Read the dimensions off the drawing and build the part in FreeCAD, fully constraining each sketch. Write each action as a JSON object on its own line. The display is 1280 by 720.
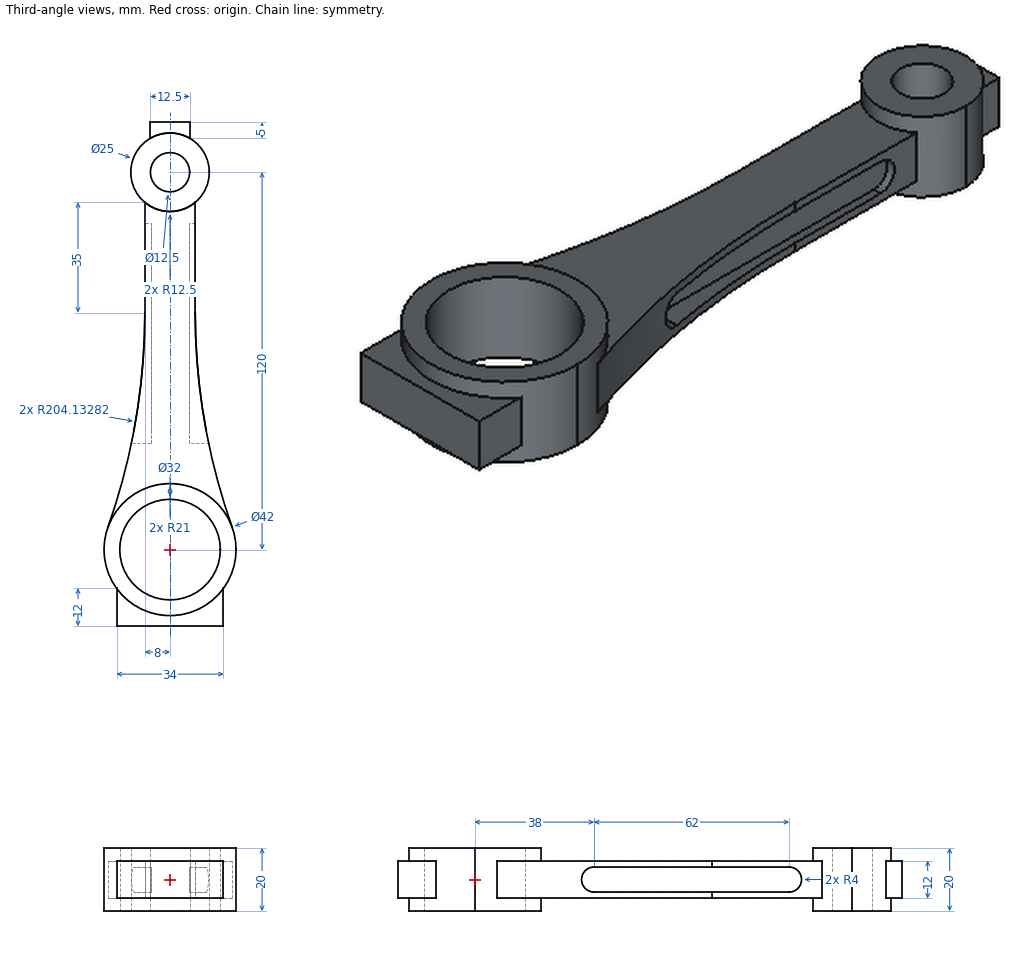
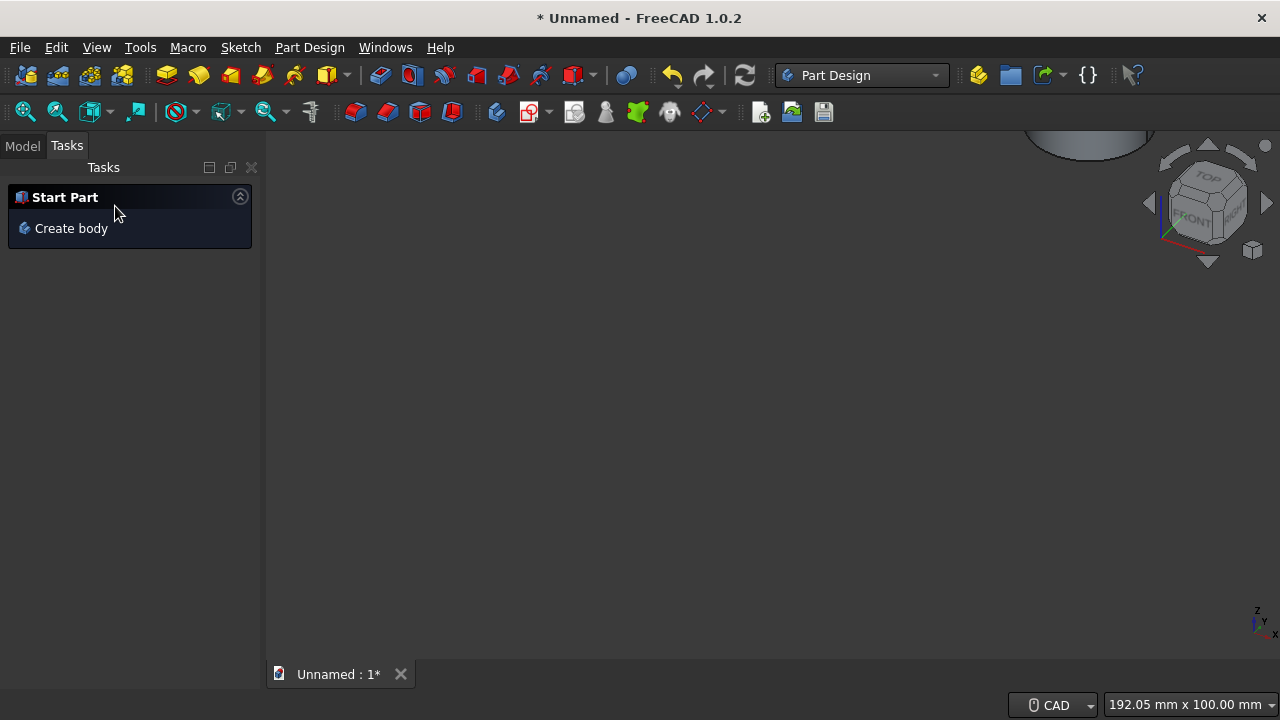
{"action": "key", "text": "v f"}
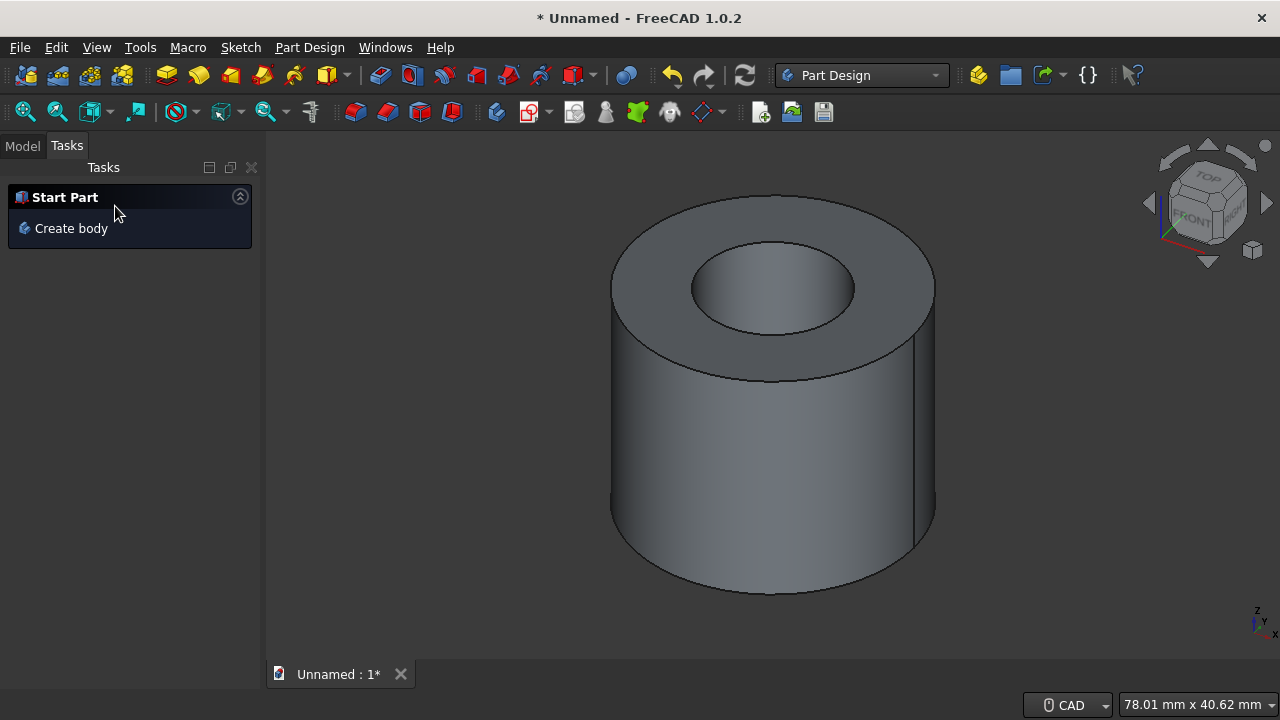
{"action": "left_click", "coordinate": [498, 112]}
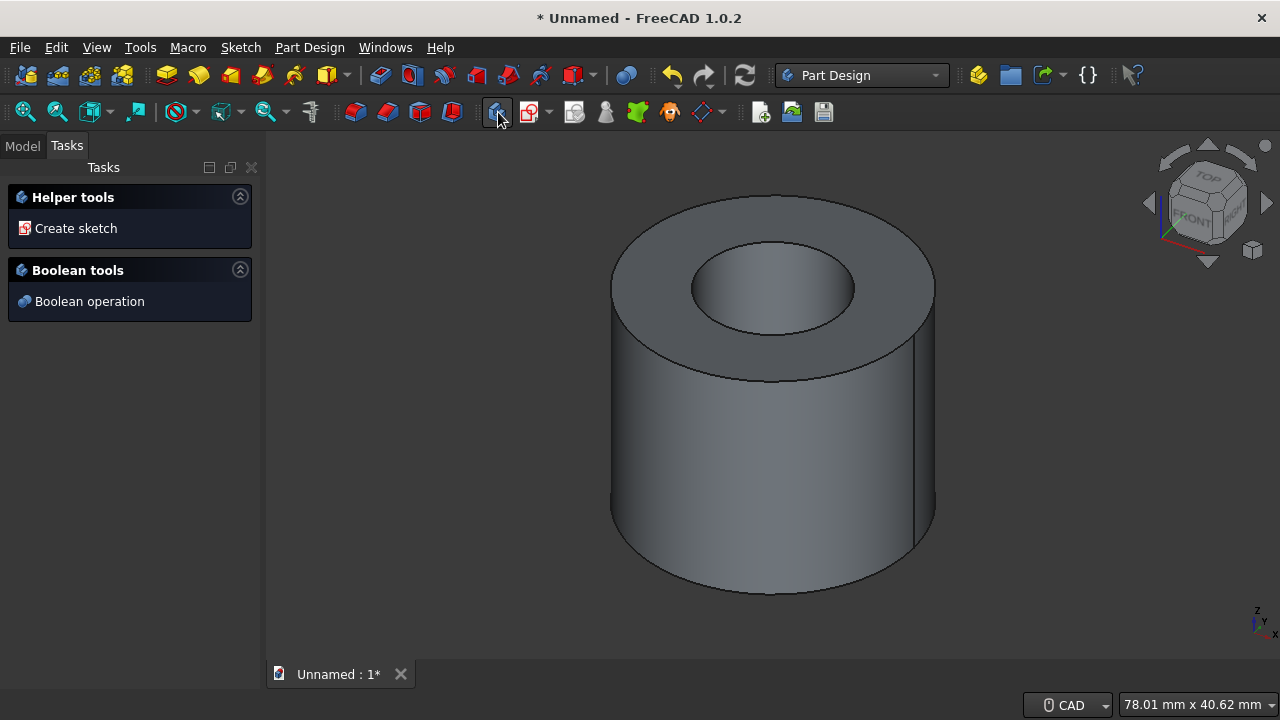
{"action": "left_click", "coordinate": [306, 619]}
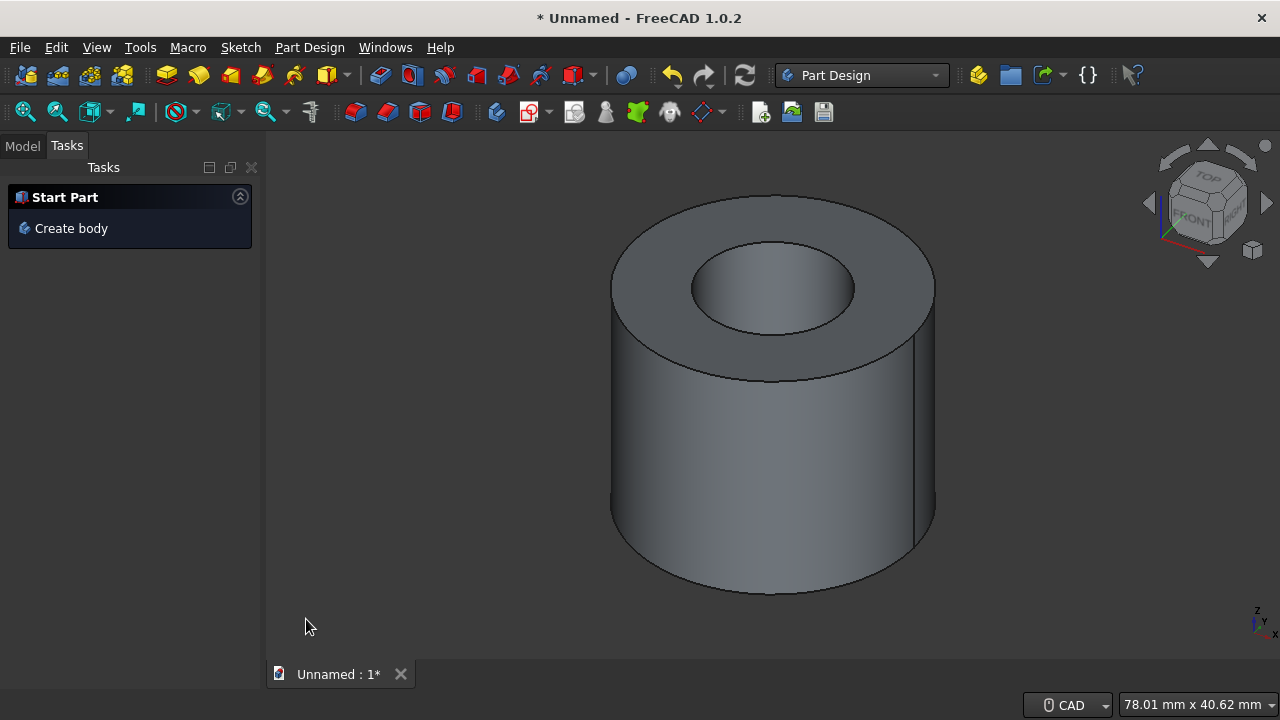
{"action": "left_click", "coordinate": [530, 112]}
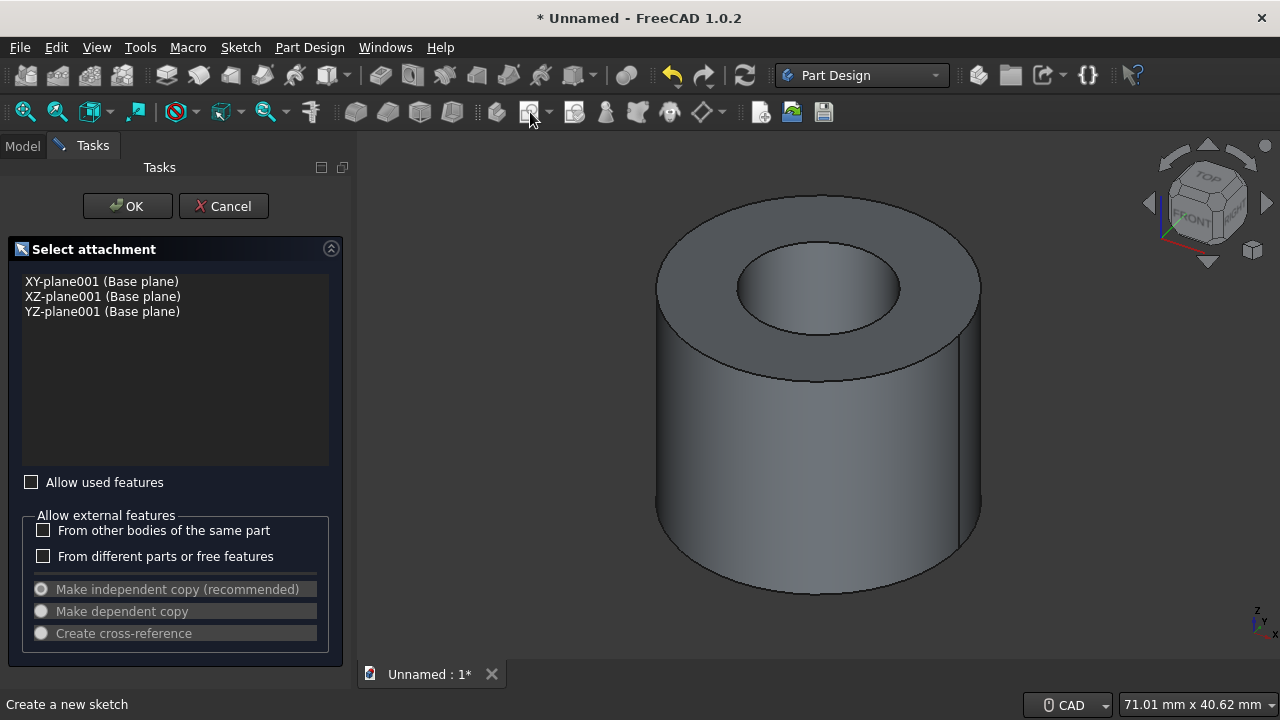
{"action": "left_click", "coordinate": [82, 282]}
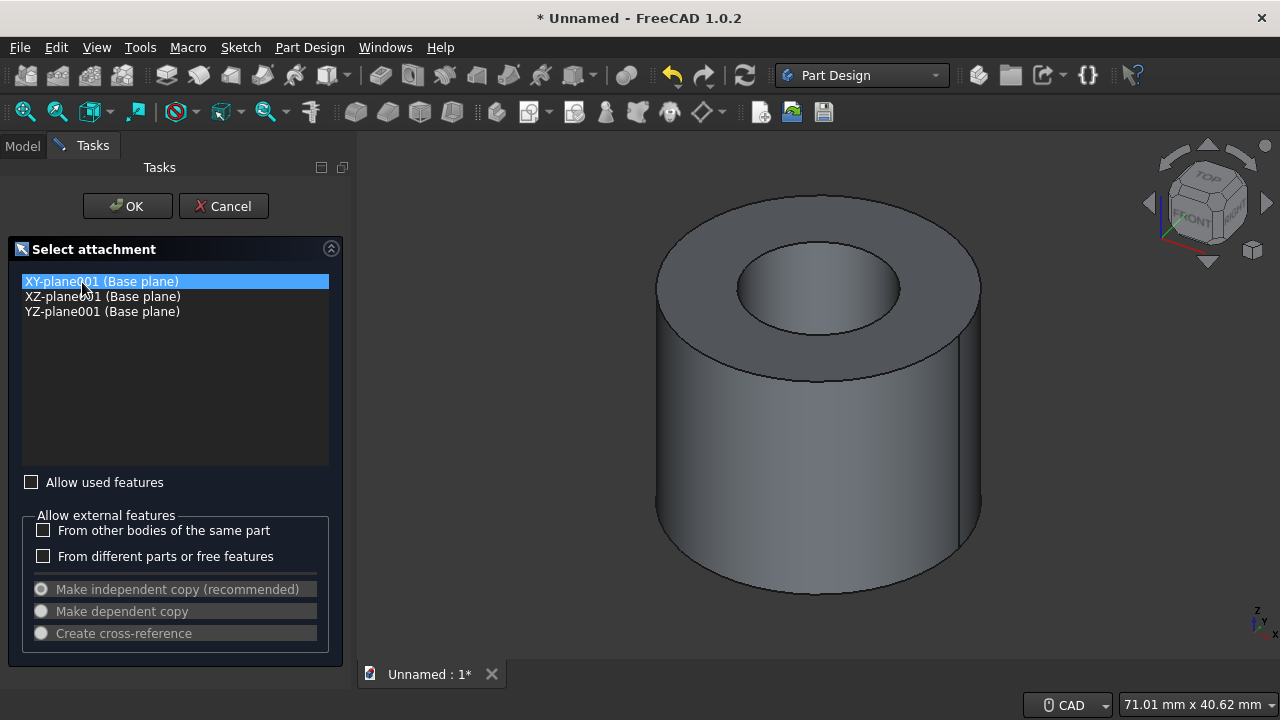
{"action": "left_click", "coordinate": [128, 206]}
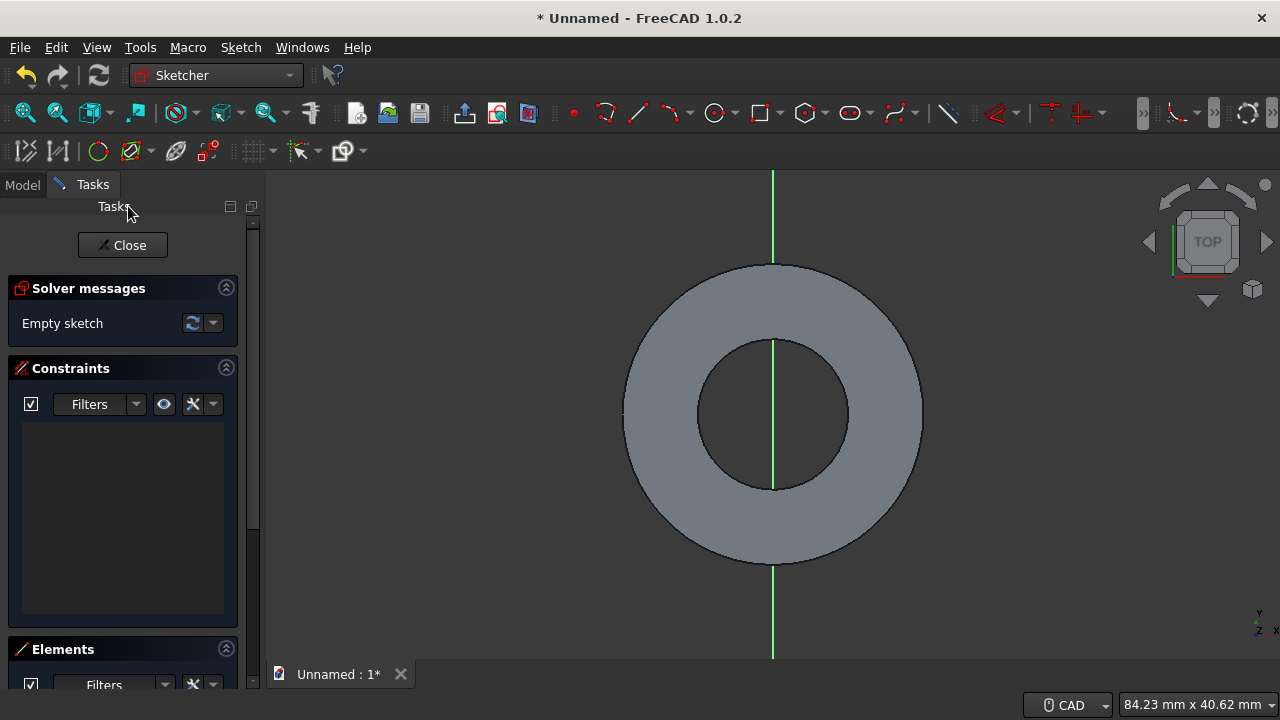
{"action": "scroll", "coordinate": [704, 414], "scroll_direction": "down", "scroll_amount": 5}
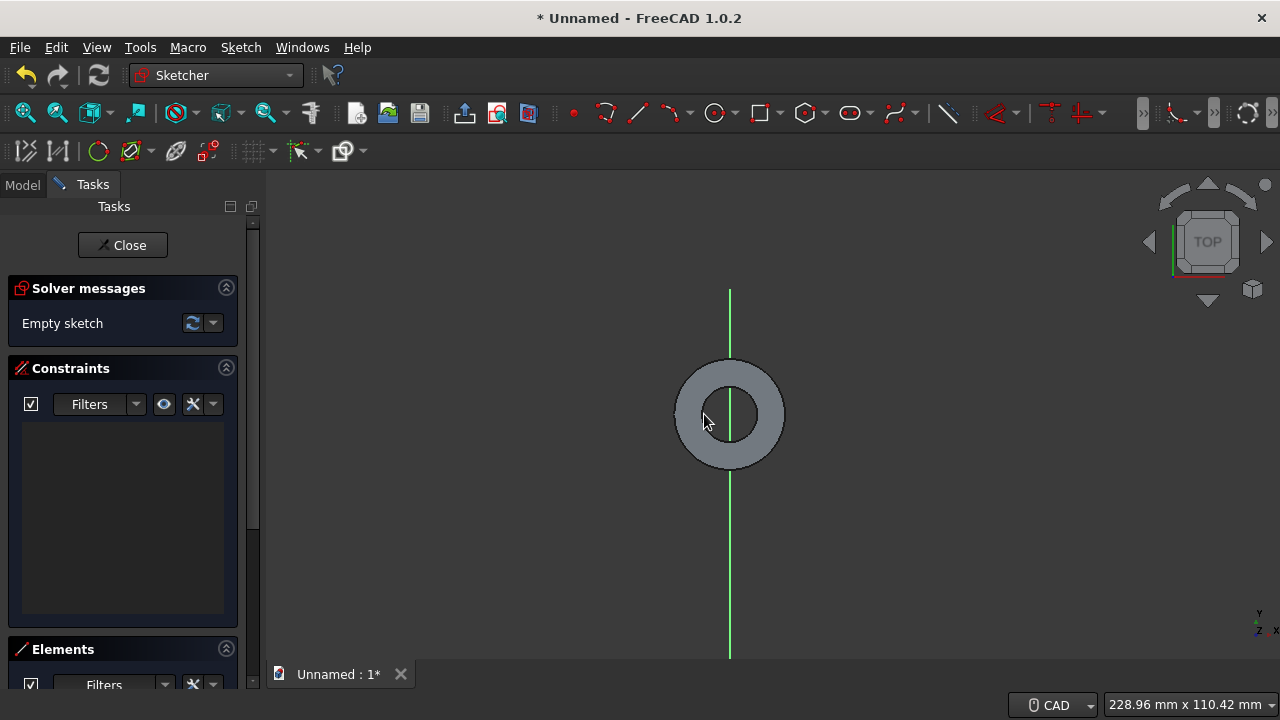
{"action": "scroll", "coordinate": [704, 414], "scroll_direction": "down", "scroll_amount": 5}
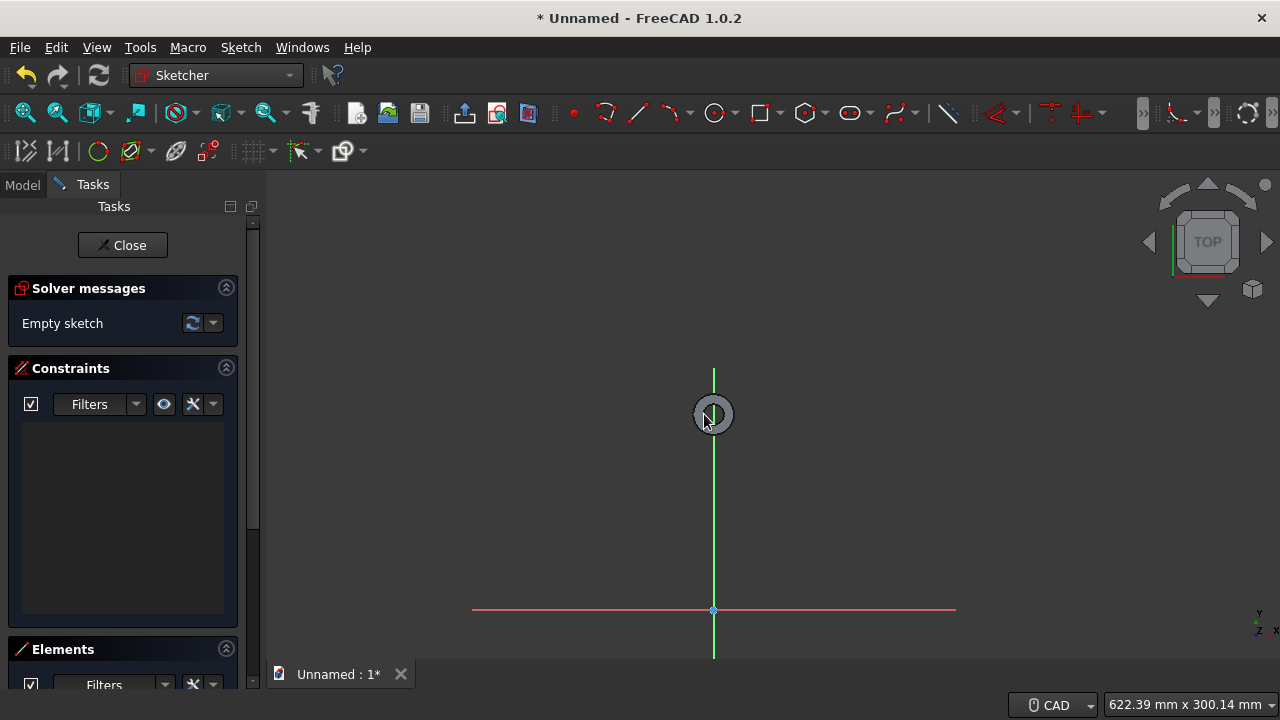
{"action": "scroll", "coordinate": [704, 414], "scroll_direction": "down", "scroll_amount": 5}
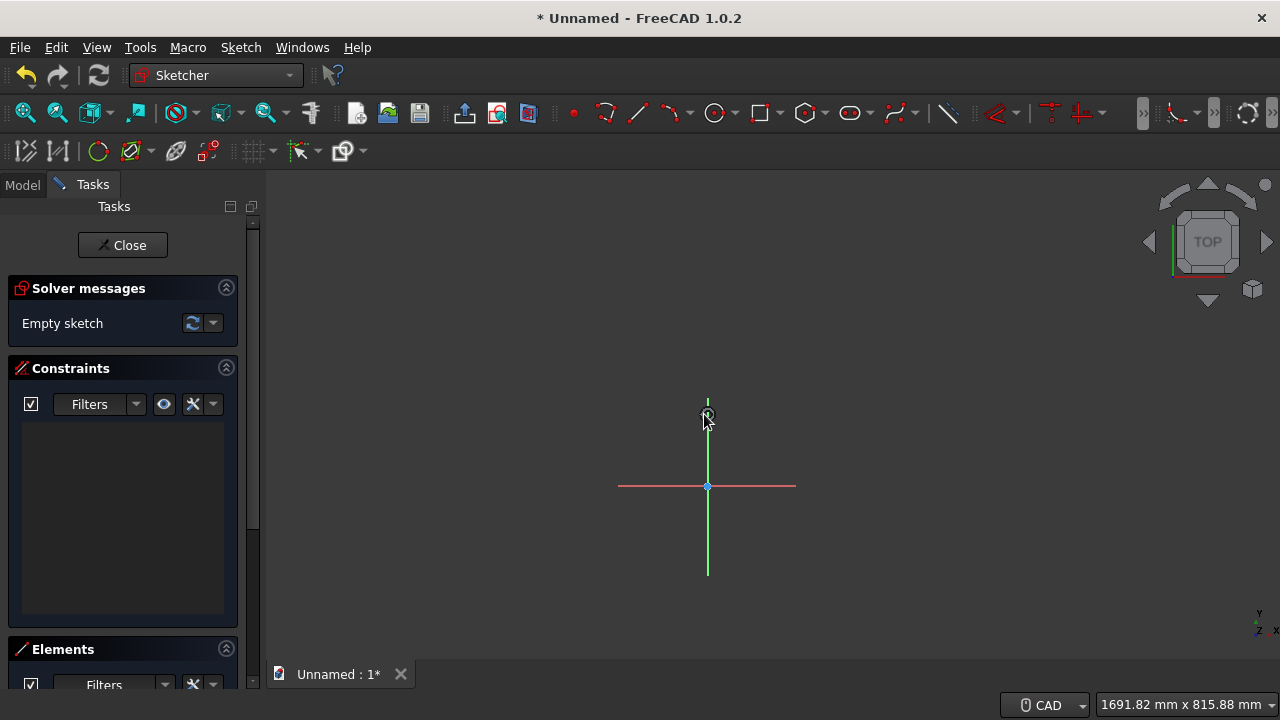
{"action": "scroll", "coordinate": [708, 494], "scroll_direction": "up", "scroll_amount": 12}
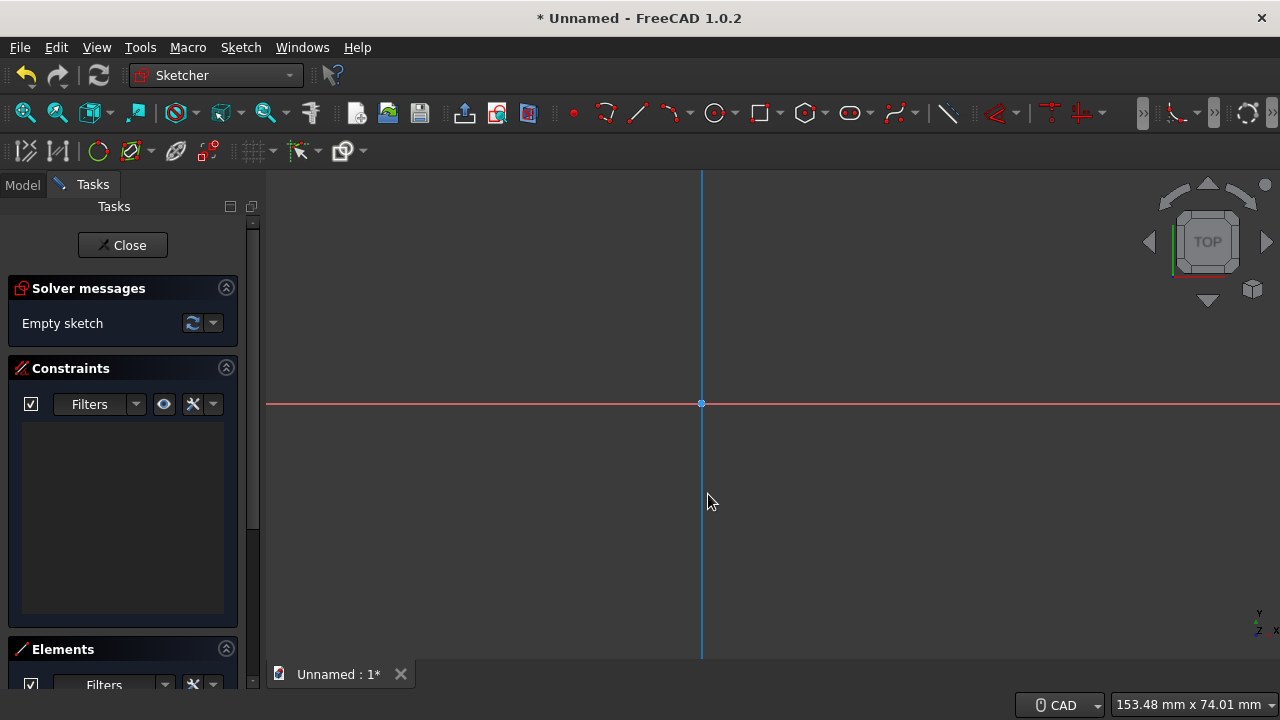
{"action": "key", "text": "g c"}